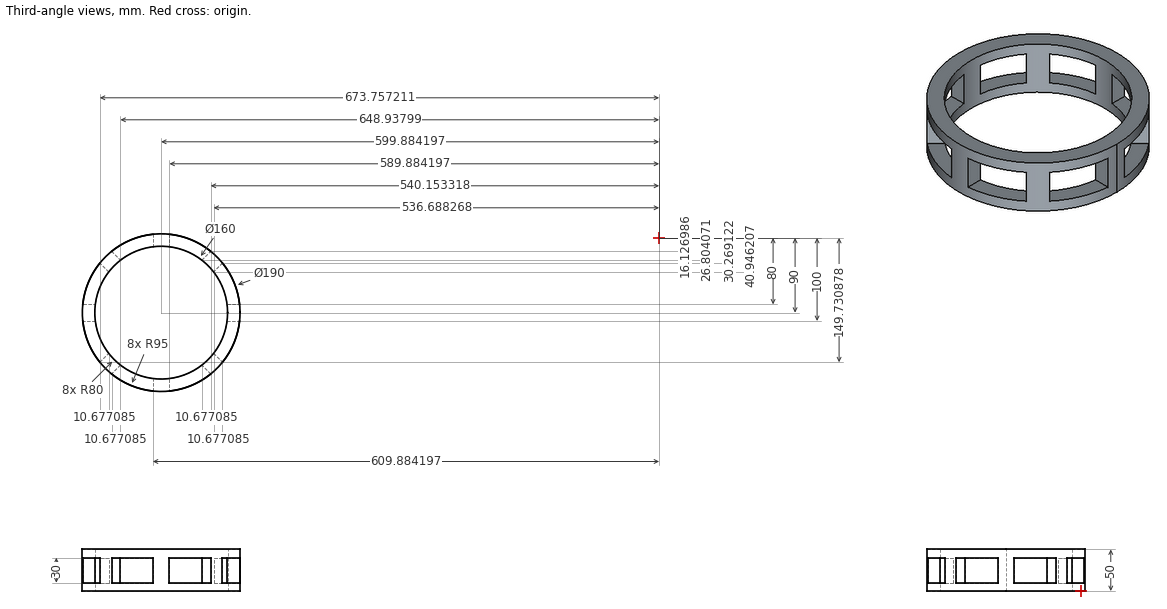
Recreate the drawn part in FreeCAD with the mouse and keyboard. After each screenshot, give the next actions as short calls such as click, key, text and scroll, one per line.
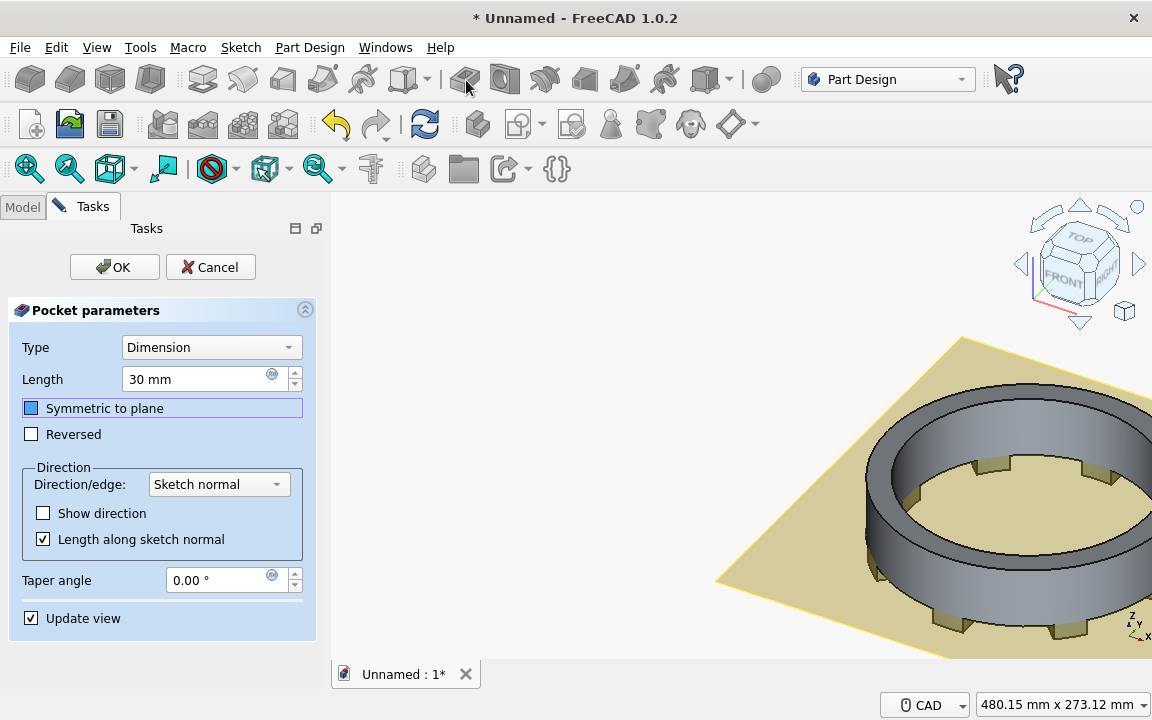
click(30, 434)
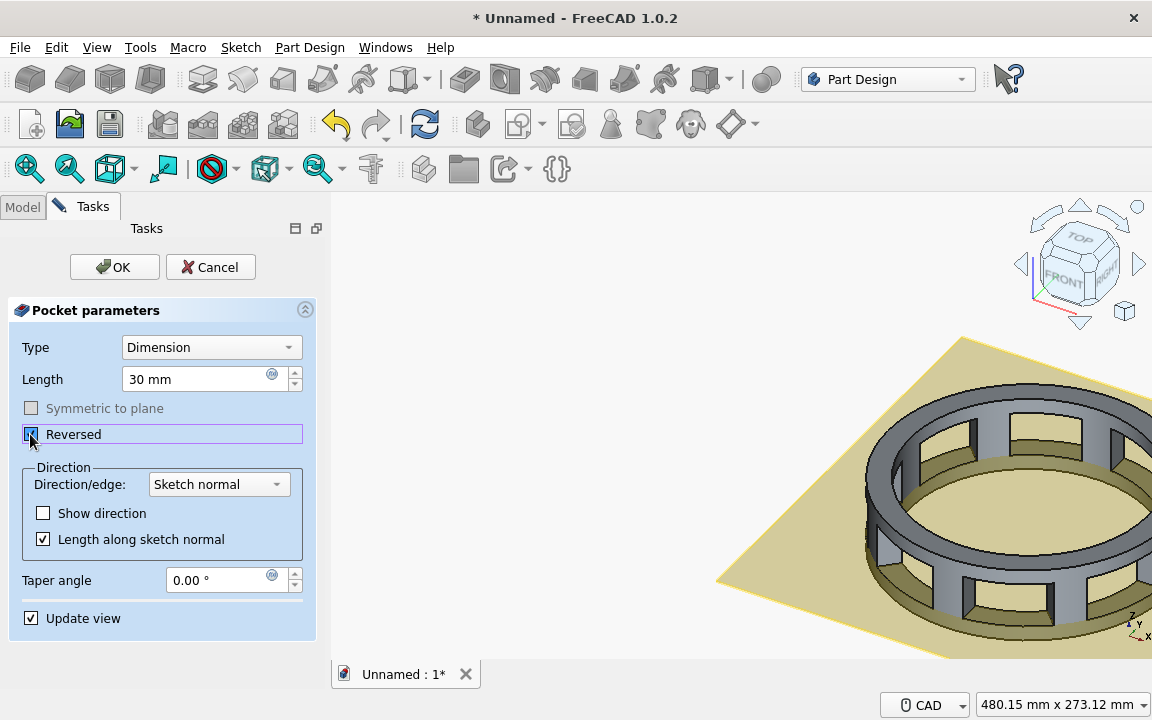
click(115, 267)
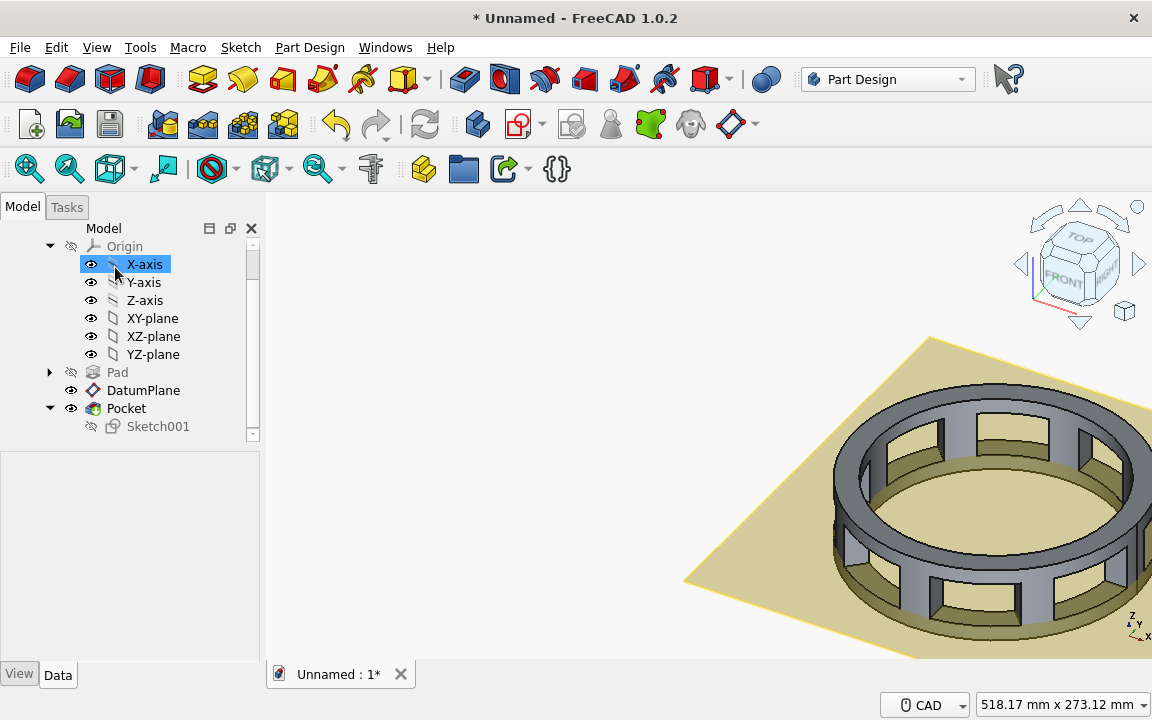
click(116, 390)
key(space)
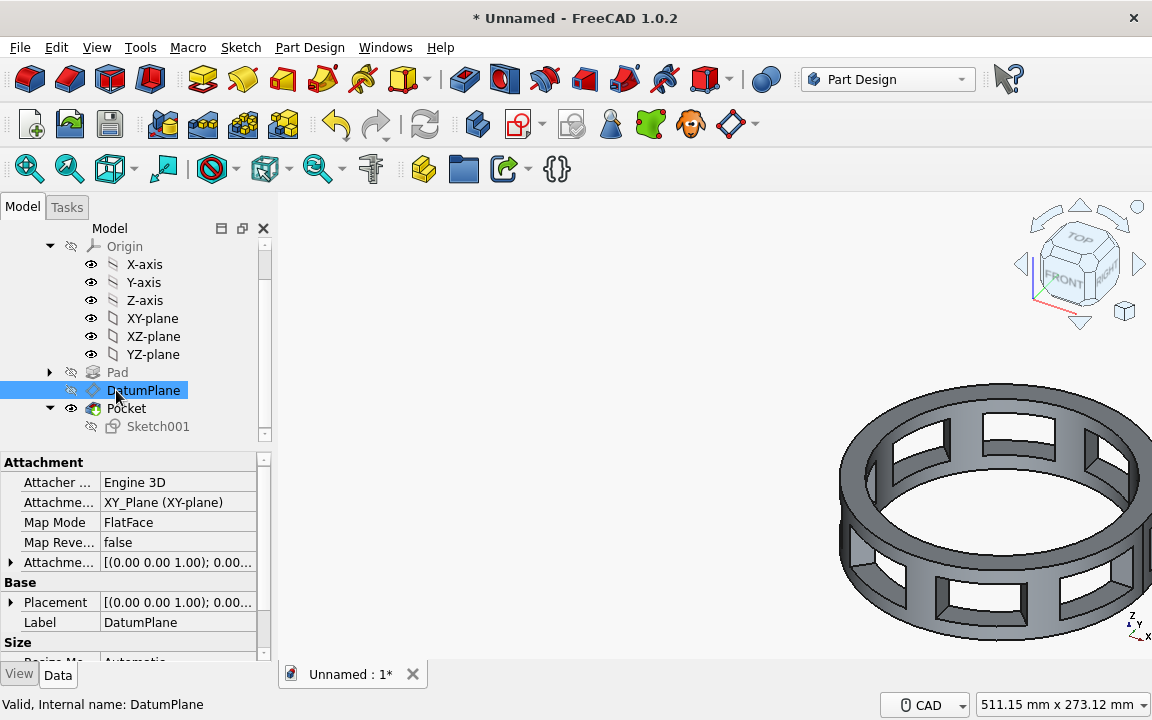
key(0)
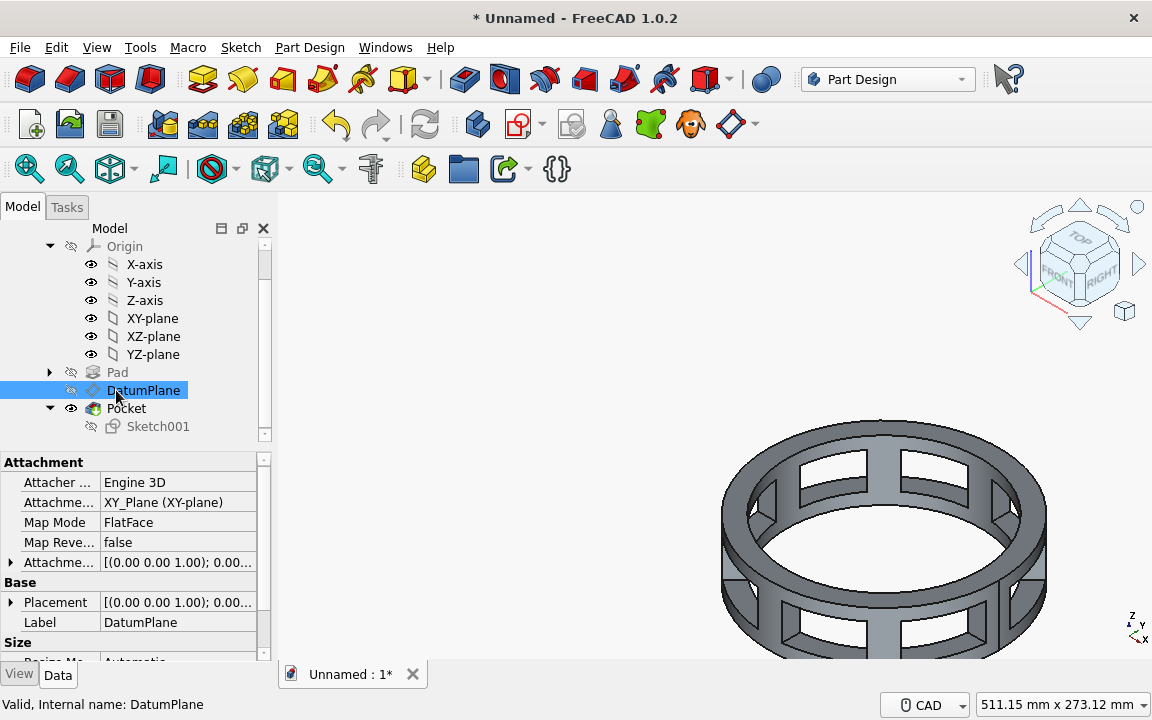
key(v)
key(f)